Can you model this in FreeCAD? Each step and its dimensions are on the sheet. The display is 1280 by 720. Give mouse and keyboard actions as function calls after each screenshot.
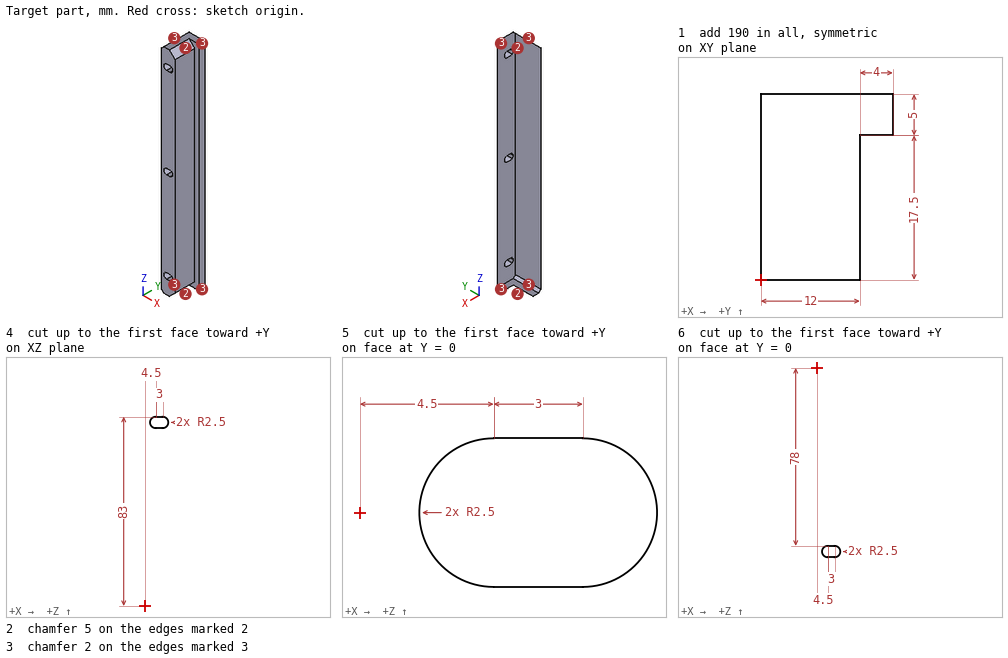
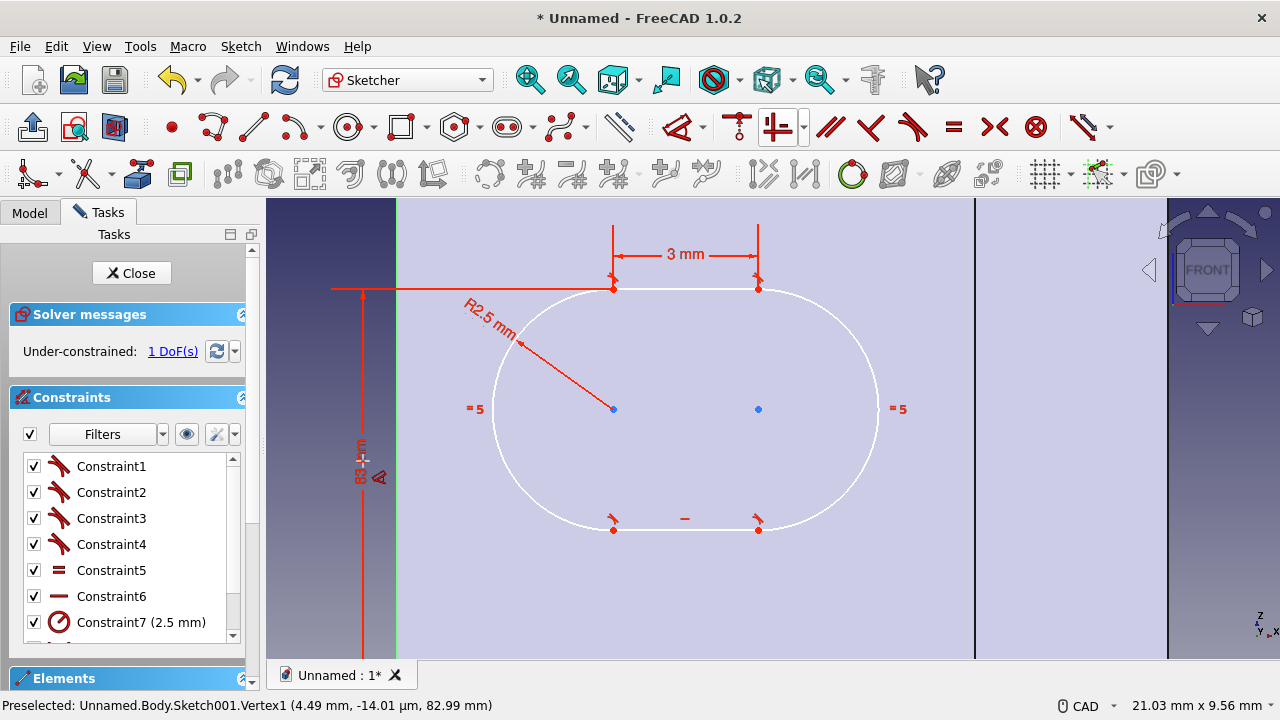
click(613, 289)
click(505, 255)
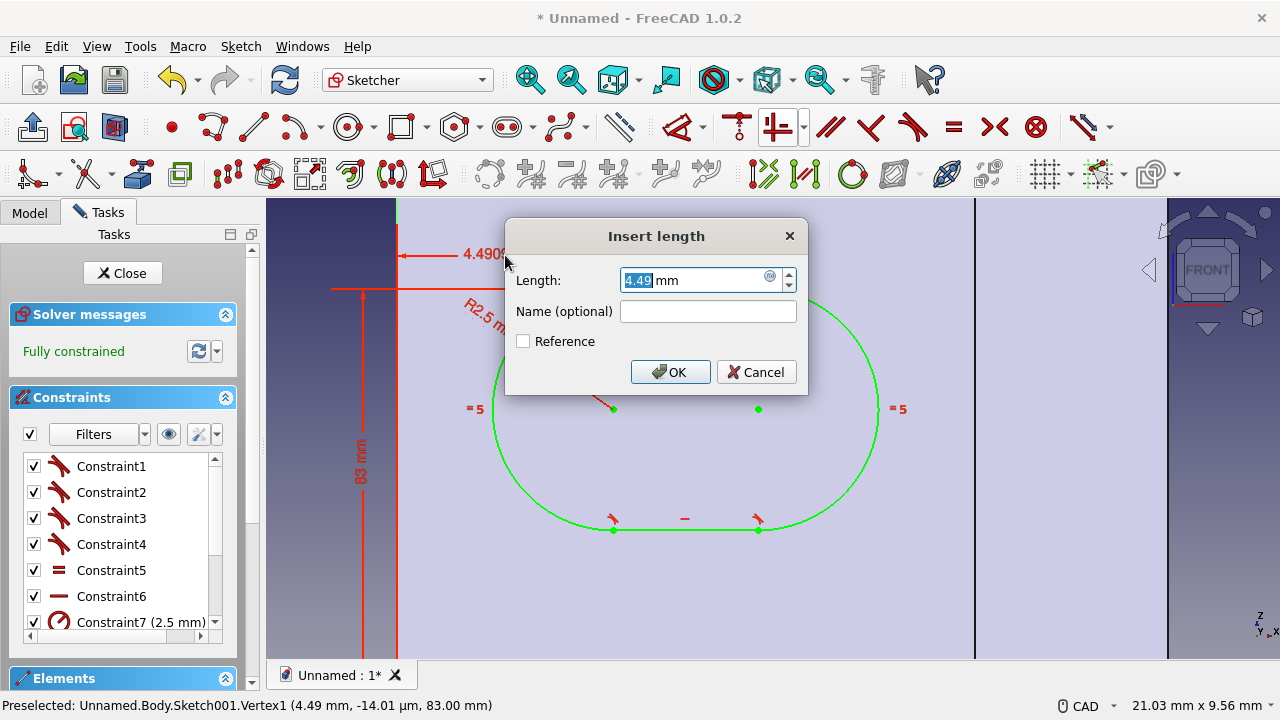
text(4.5)
key(Return)
key(Escape)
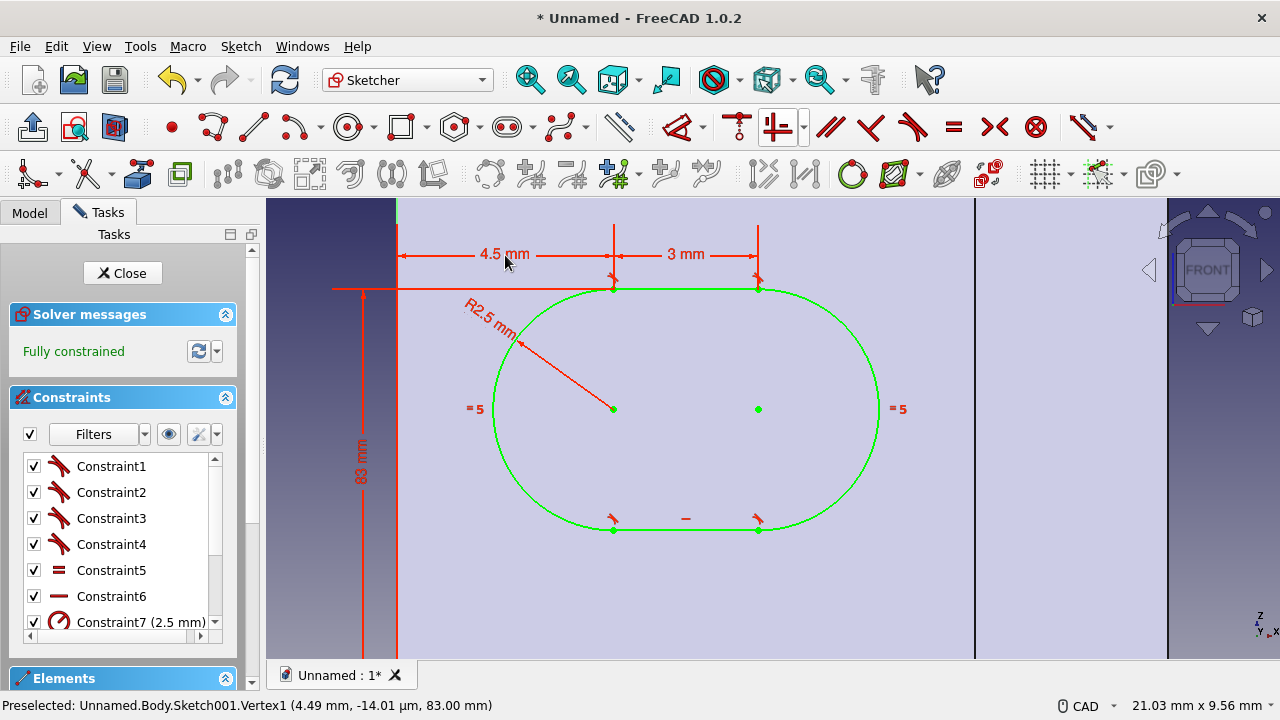
click(123, 273)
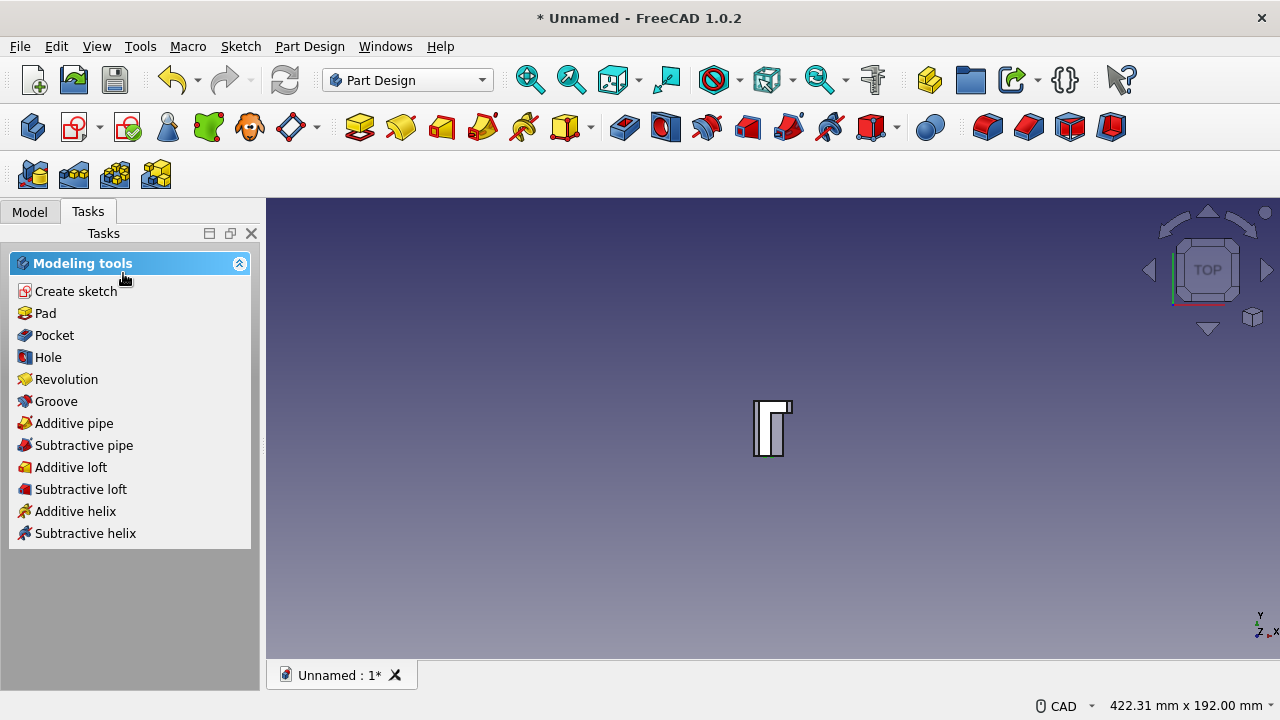
click(625, 128)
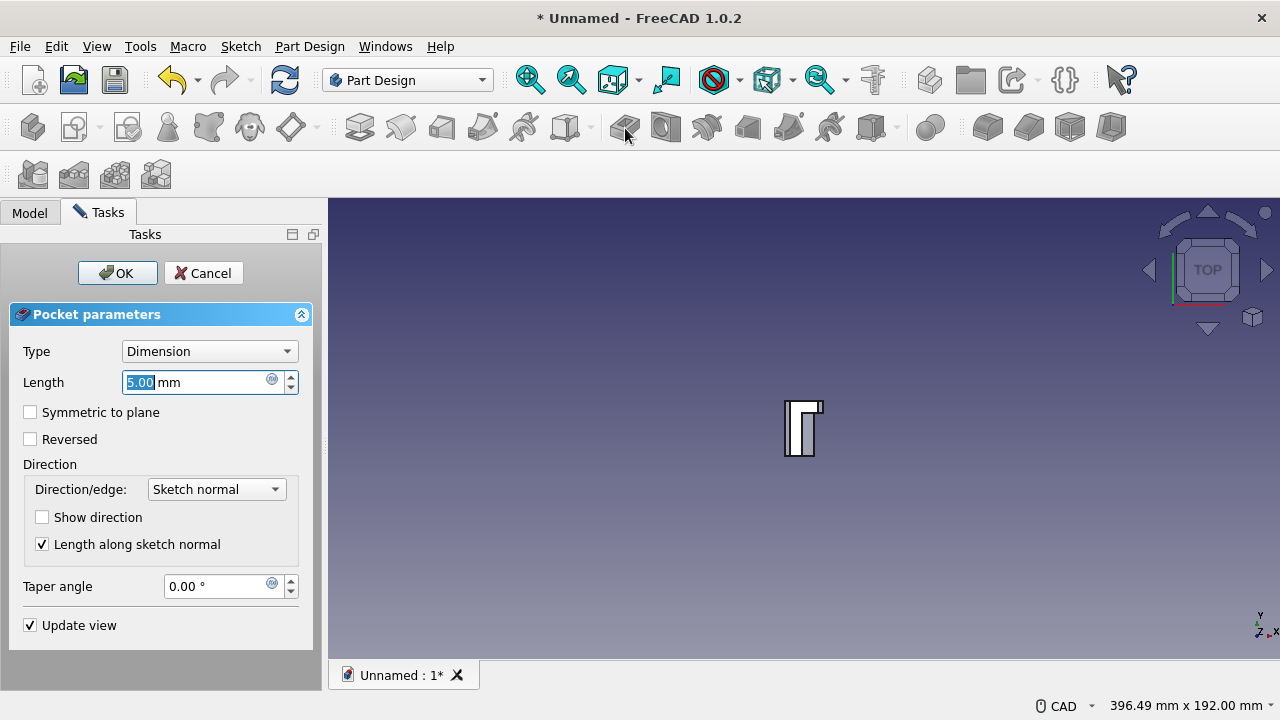
click(210, 352)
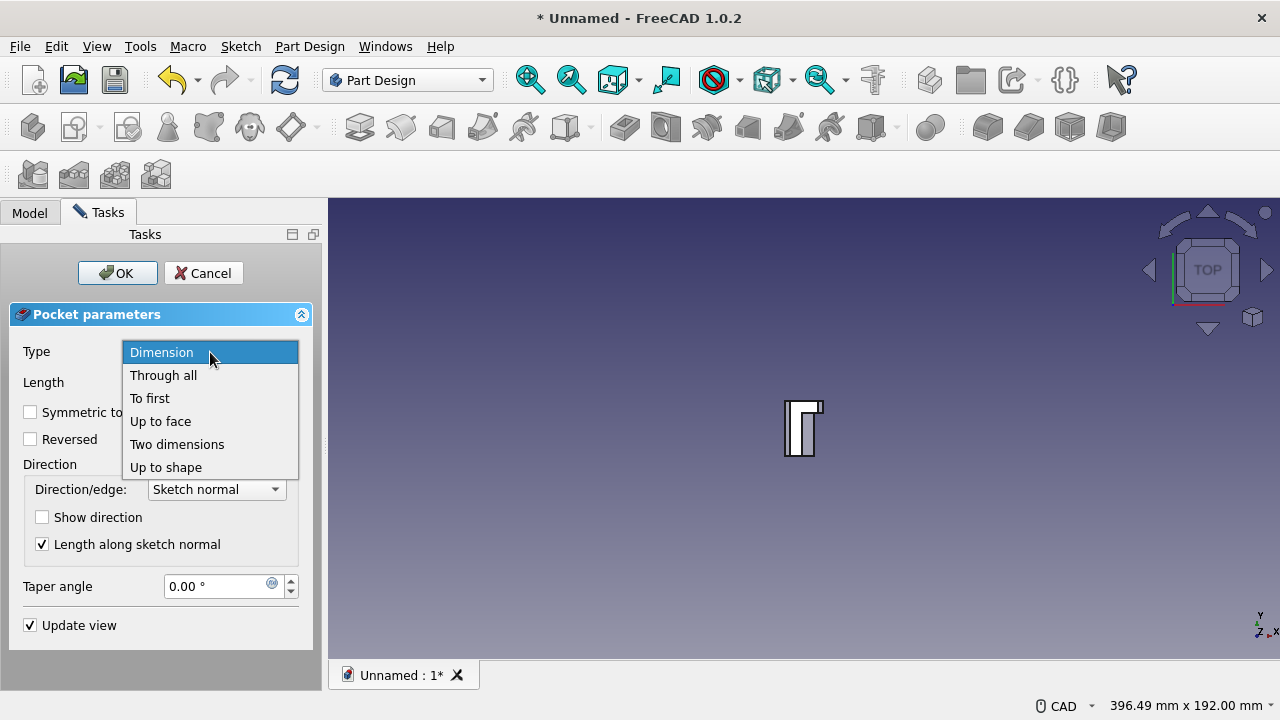
click(208, 398)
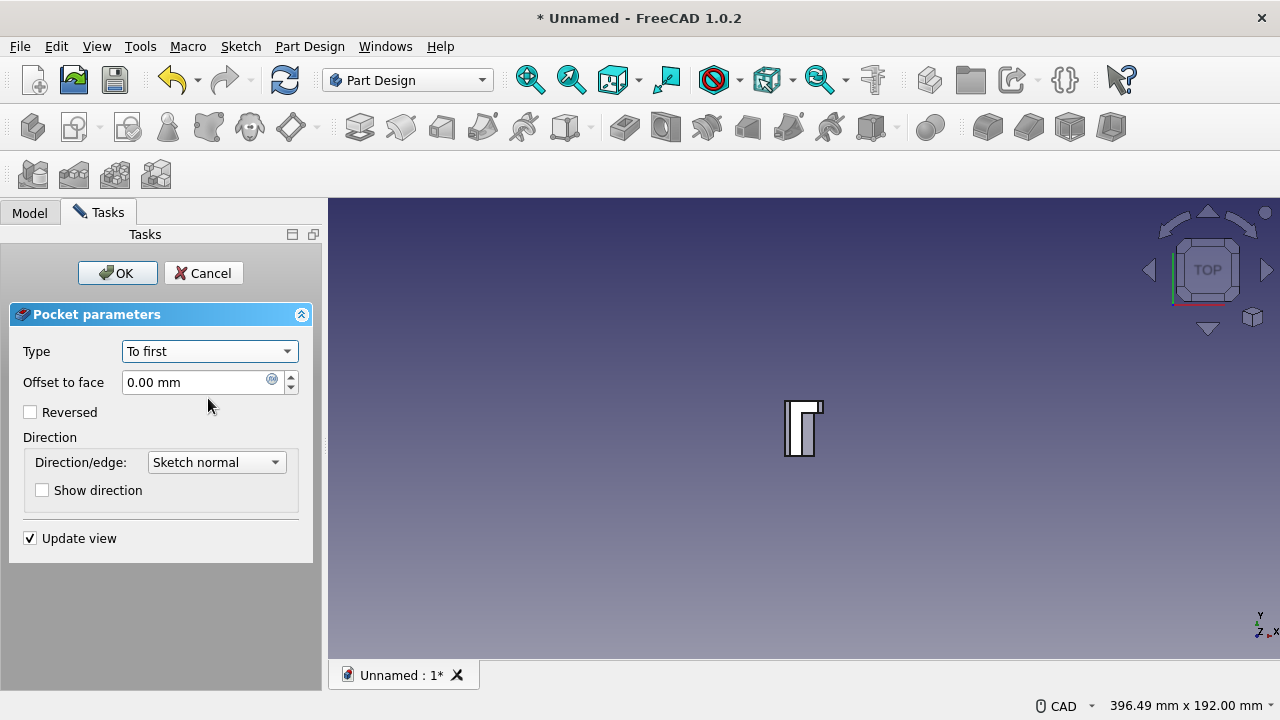
click(118, 273)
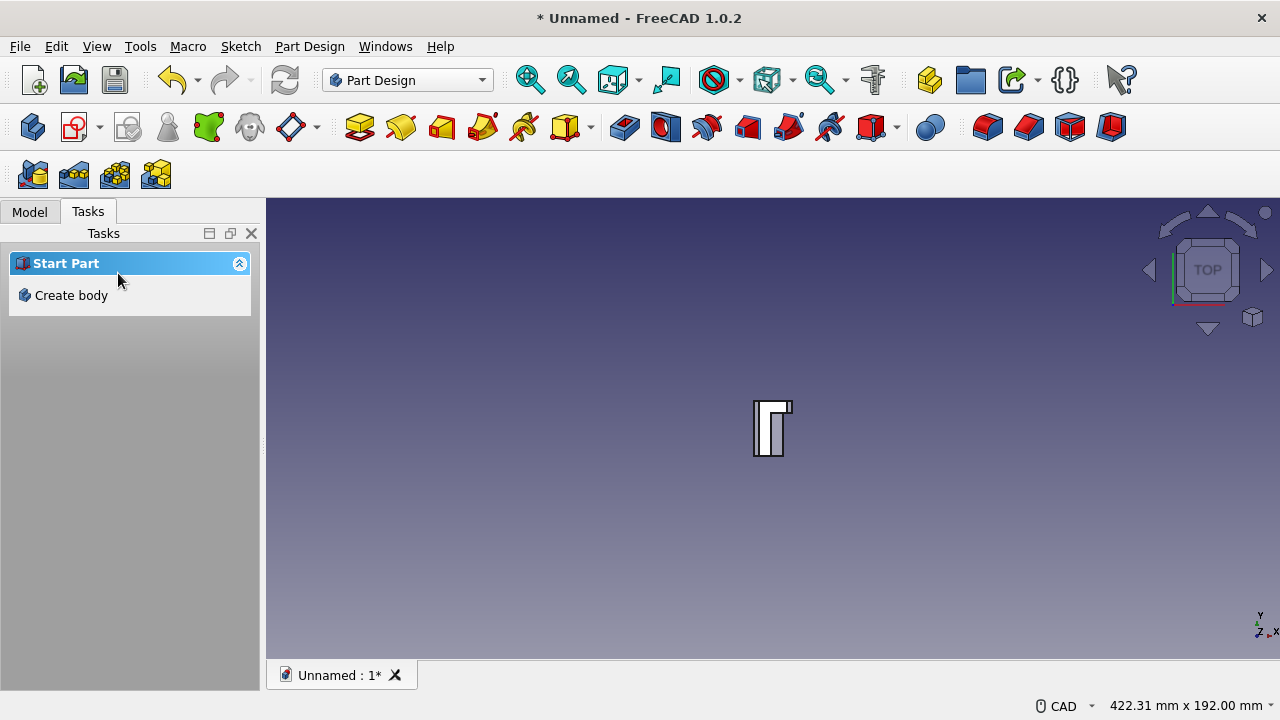
click(531, 80)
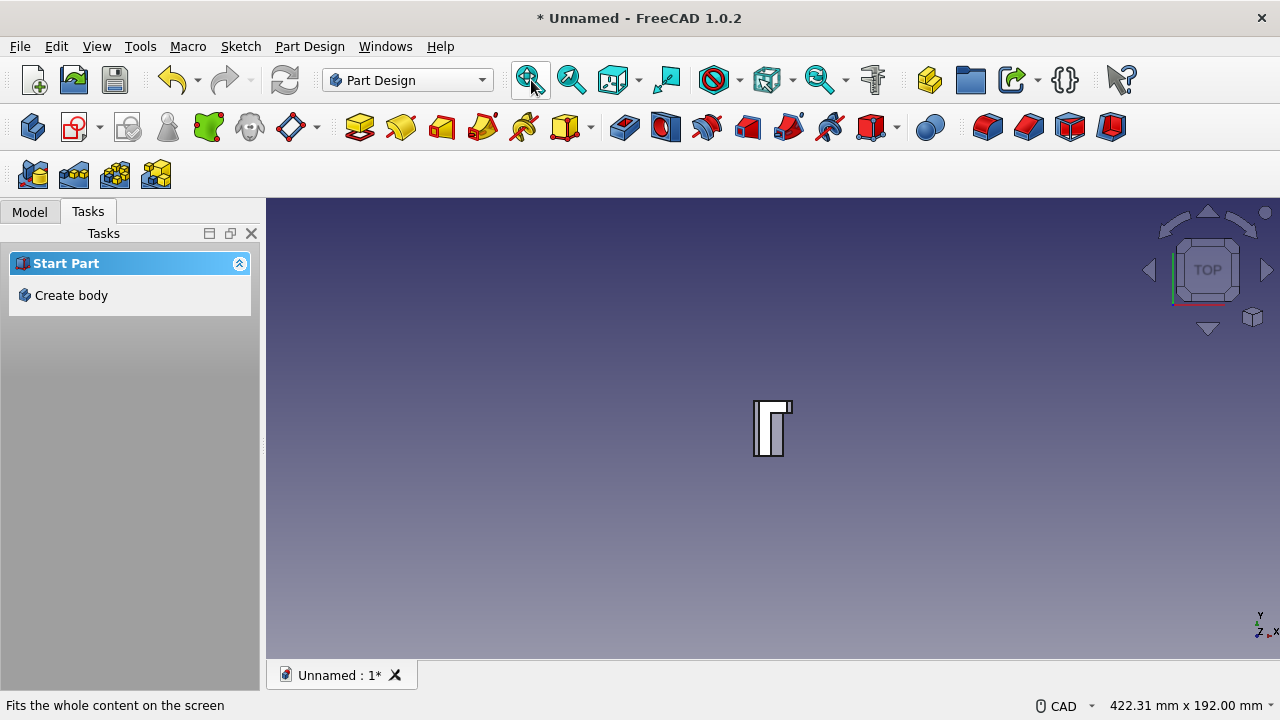
key(0)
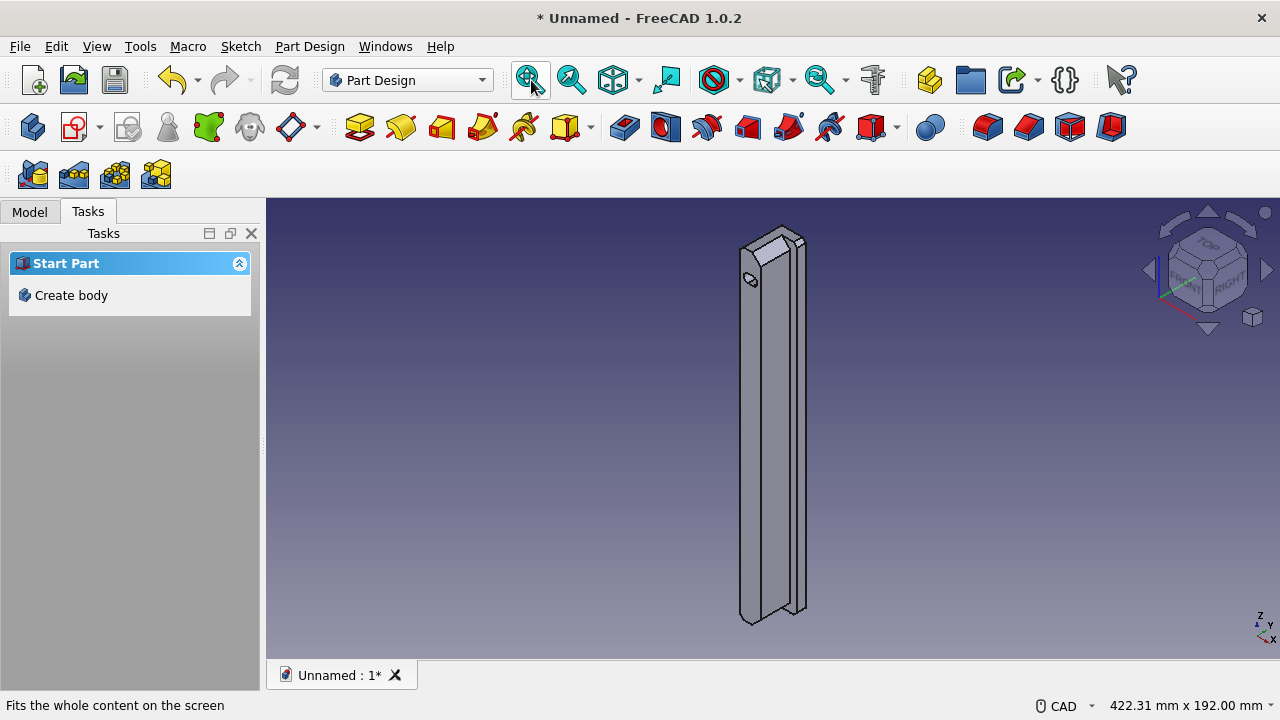
click(751, 330)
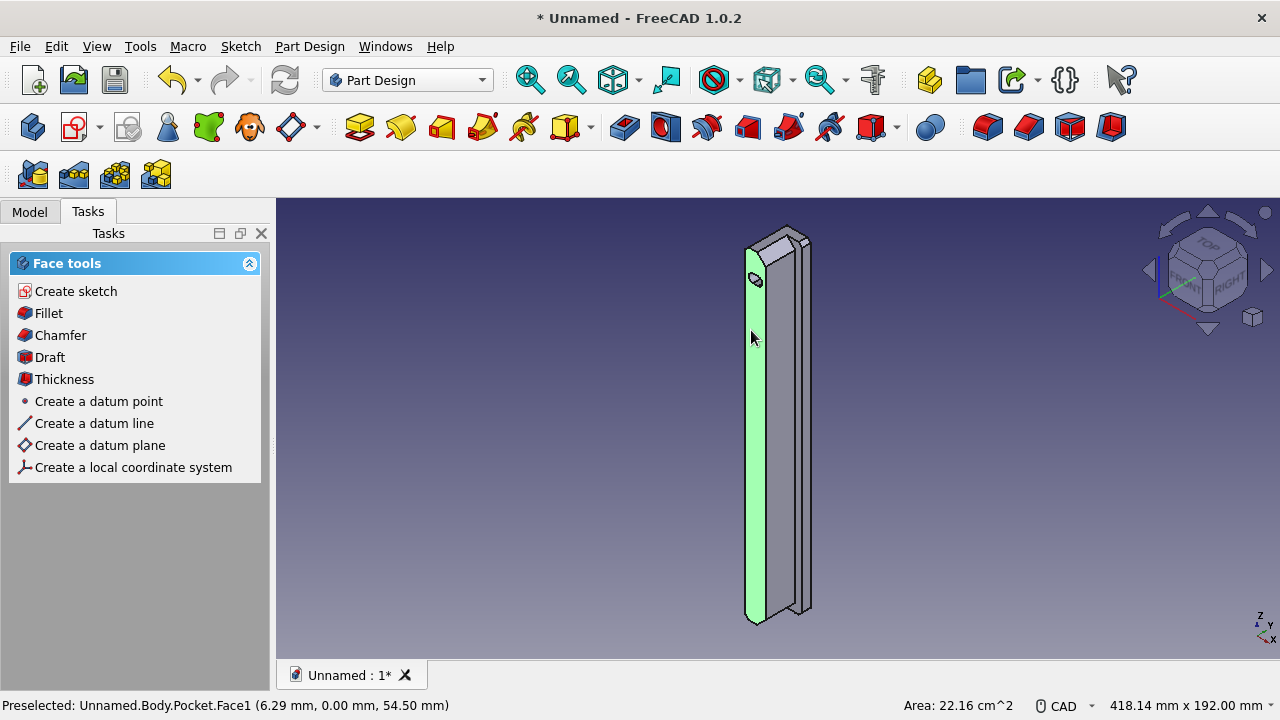
click(74, 128)